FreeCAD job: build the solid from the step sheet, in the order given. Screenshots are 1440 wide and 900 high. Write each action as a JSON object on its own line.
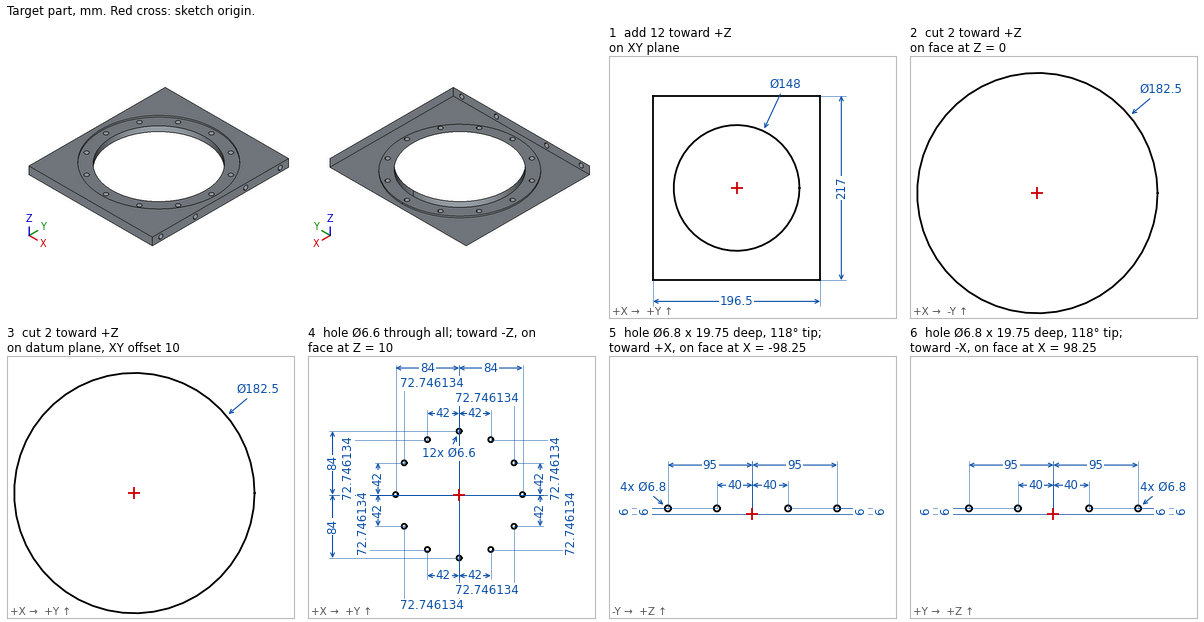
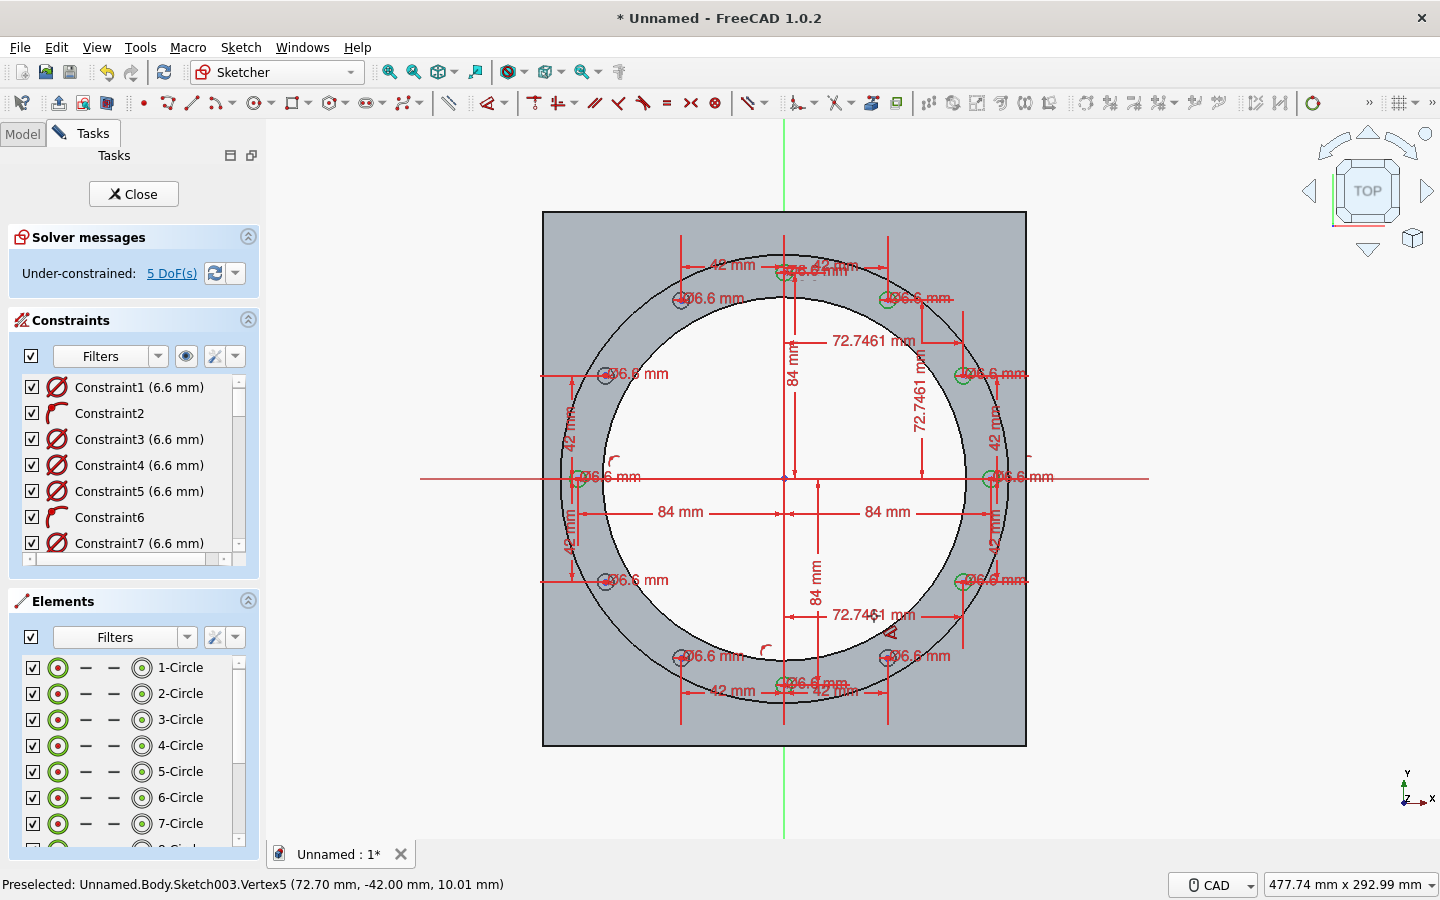
{"action": "left_click", "coordinate": [888, 658]}
{"action": "left_click", "coordinate": [922, 569]}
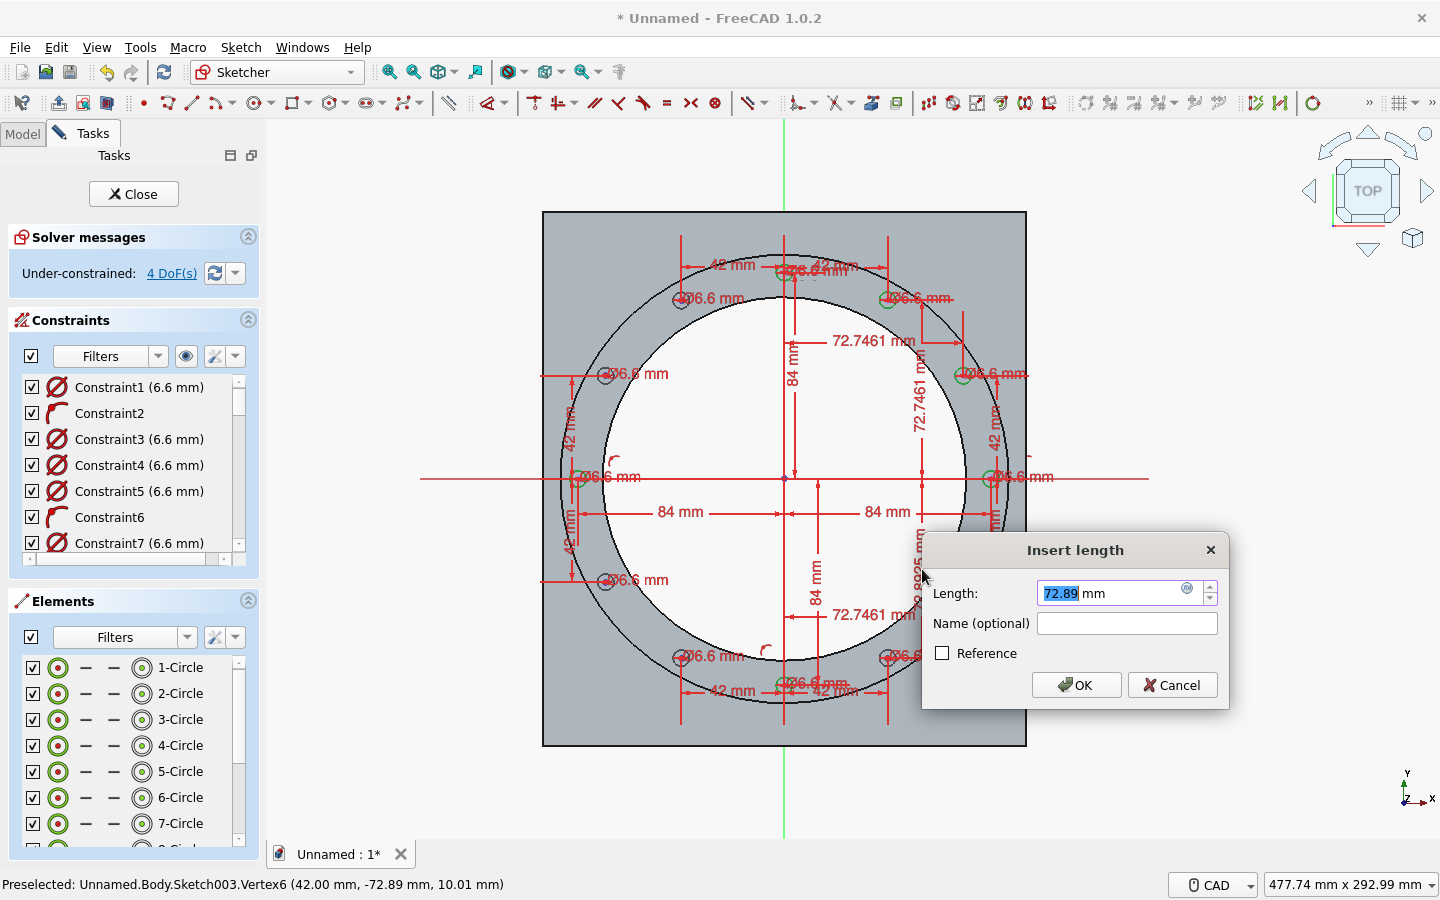
{"action": "type", "text": "72.746134"}
{"action": "key", "text": "Return"}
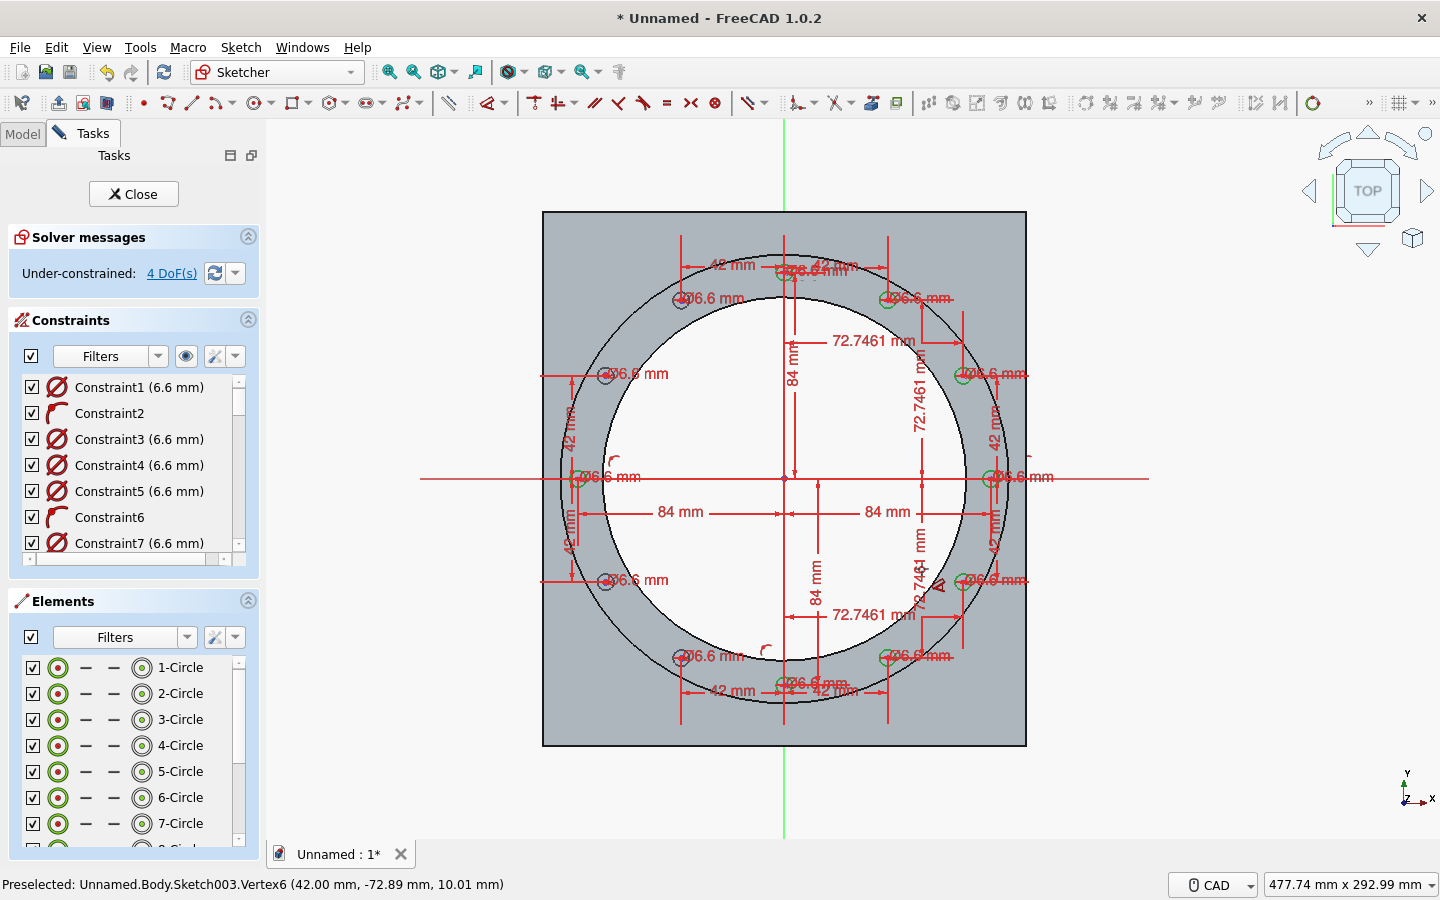
{"action": "left_click", "coordinate": [681, 658]}
{"action": "left_click", "coordinate": [647, 569]}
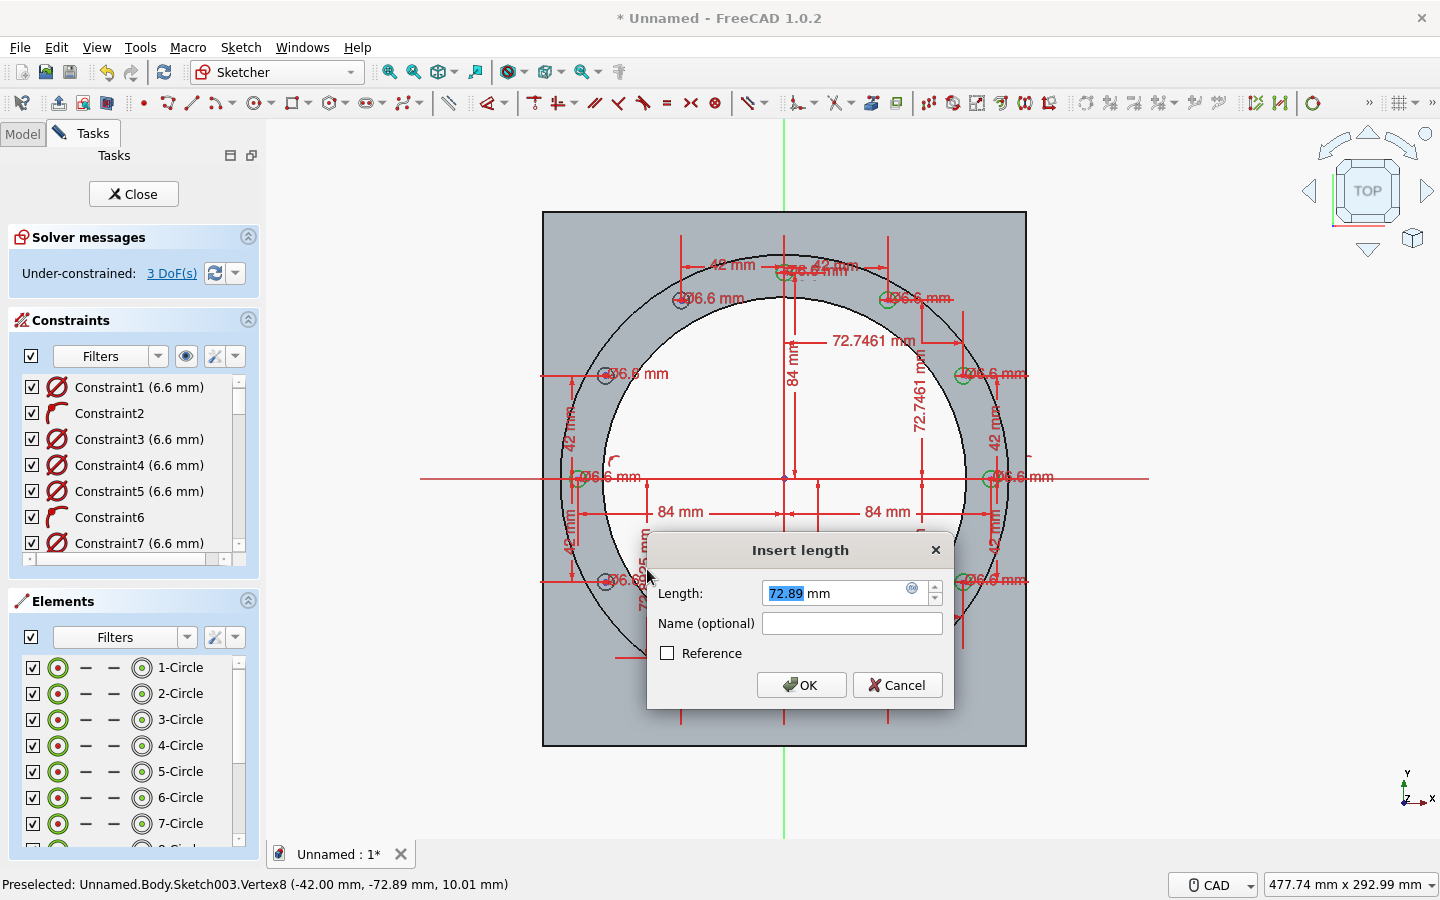
{"action": "type", "text": "72.746134"}
{"action": "key", "text": "Return"}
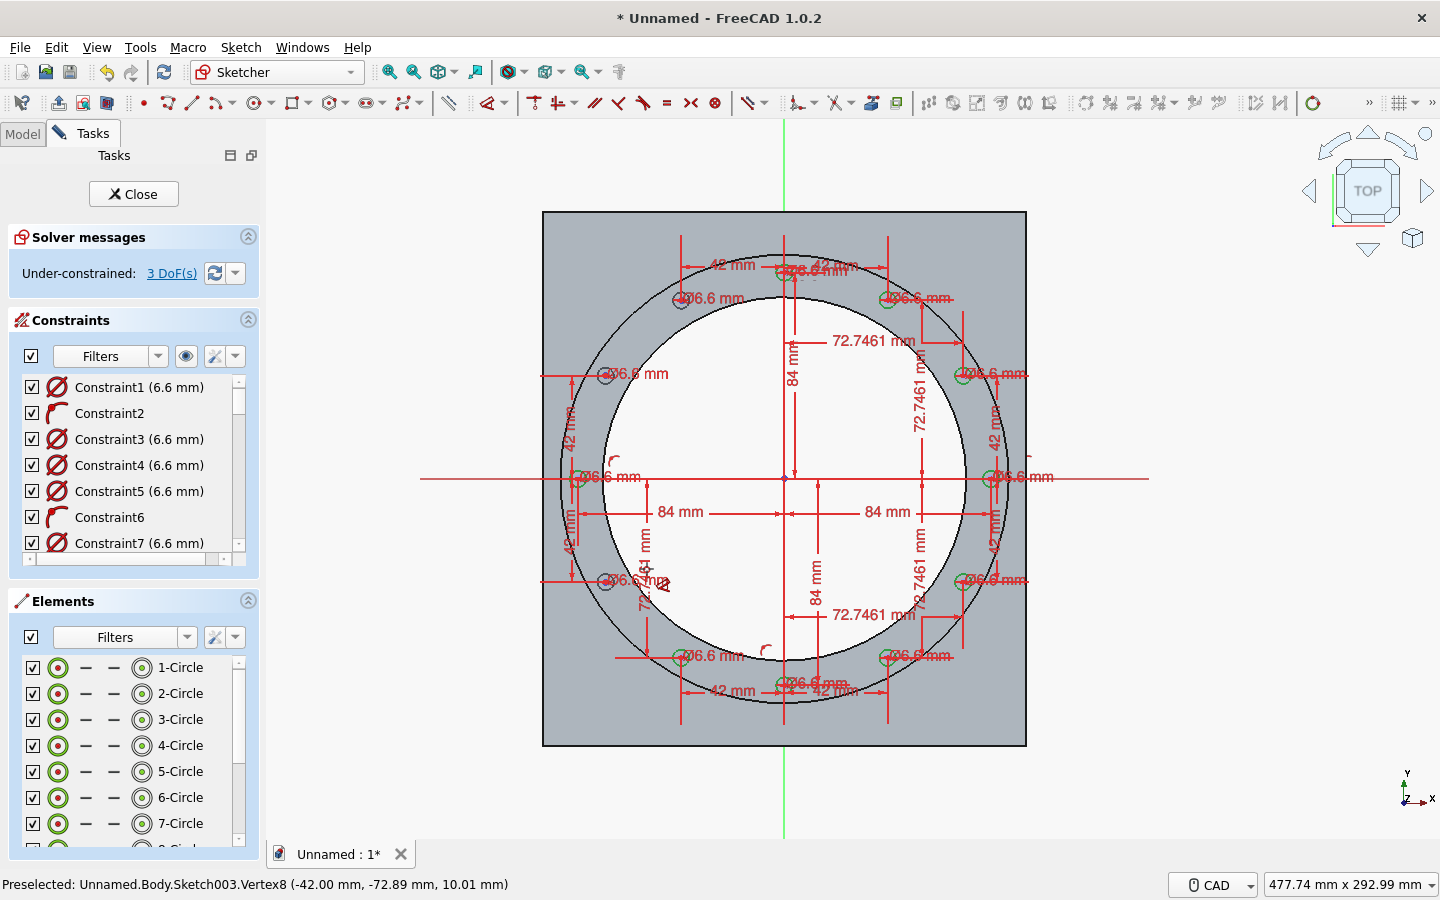
{"action": "left_click", "coordinate": [606, 582]}
{"action": "left_click", "coordinate": [695, 616]}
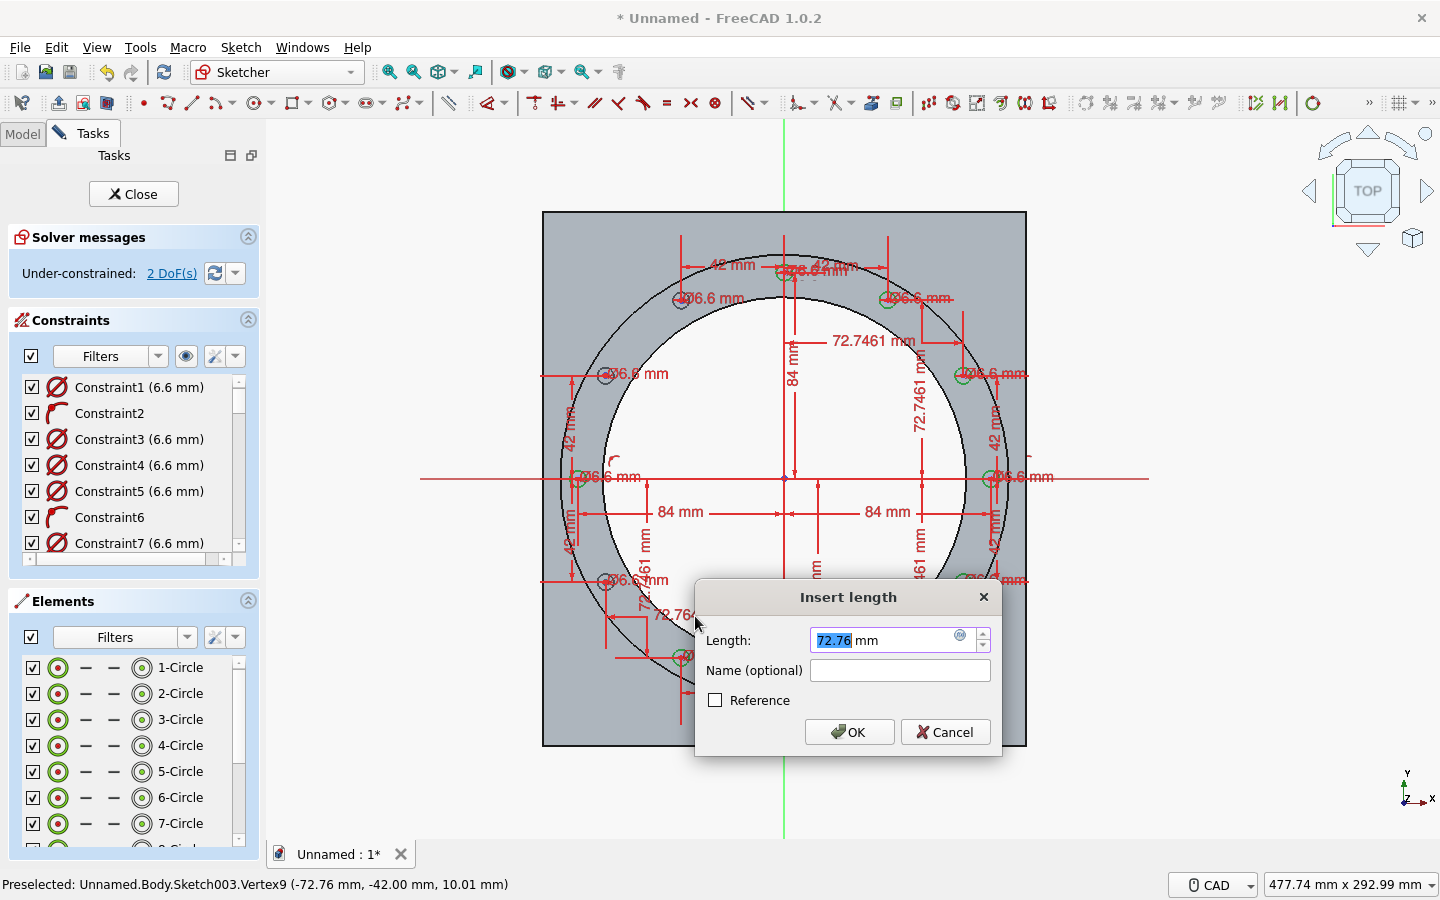
{"action": "type", "text": "72.746134"}
{"action": "key", "text": "Return"}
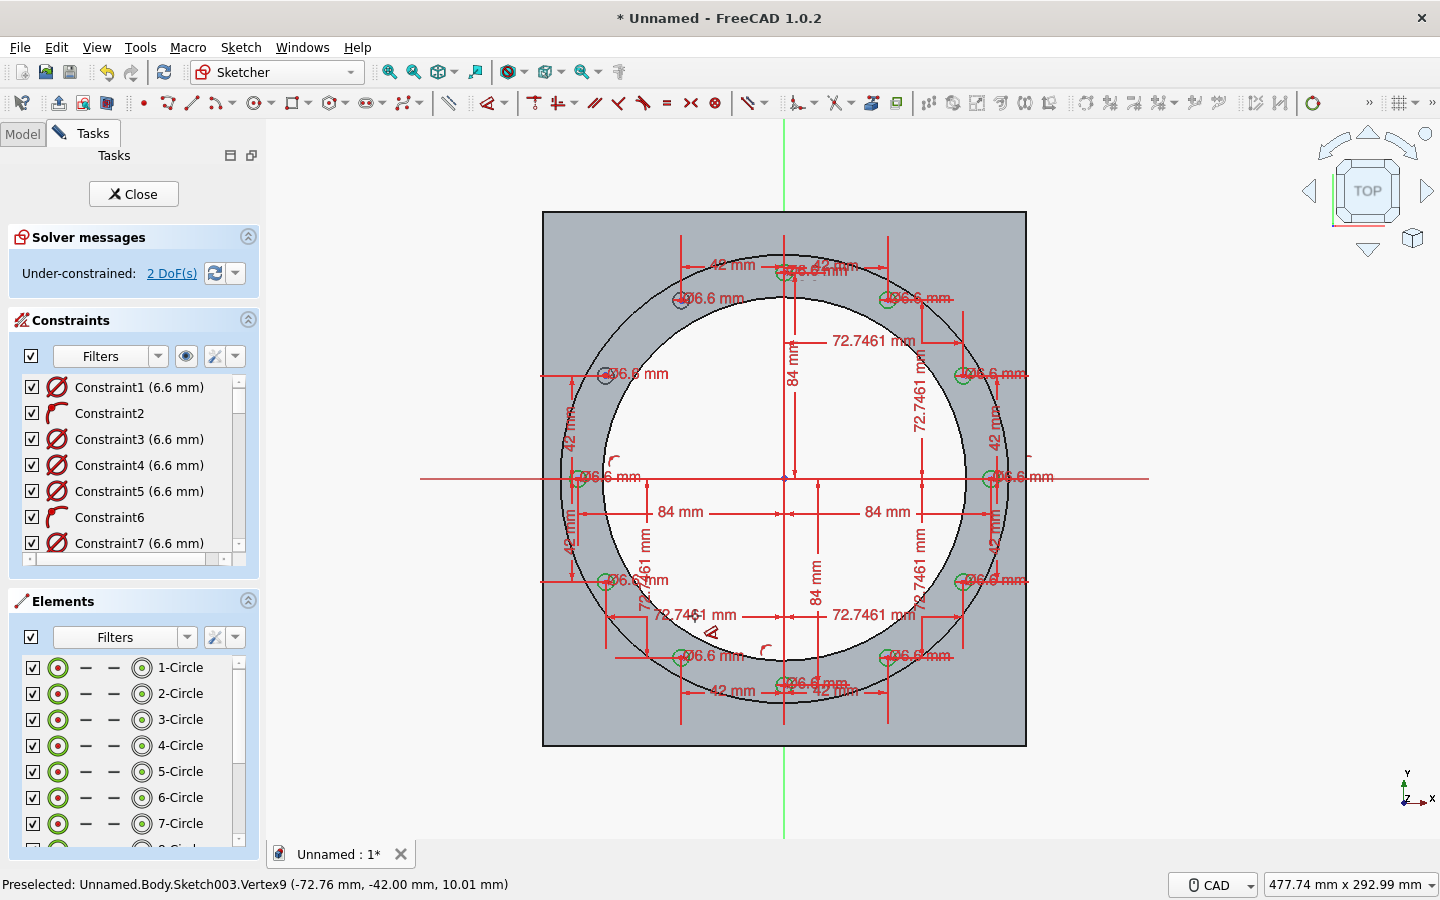
{"action": "left_click", "coordinate": [606, 376]}
{"action": "left_click", "coordinate": [695, 342]}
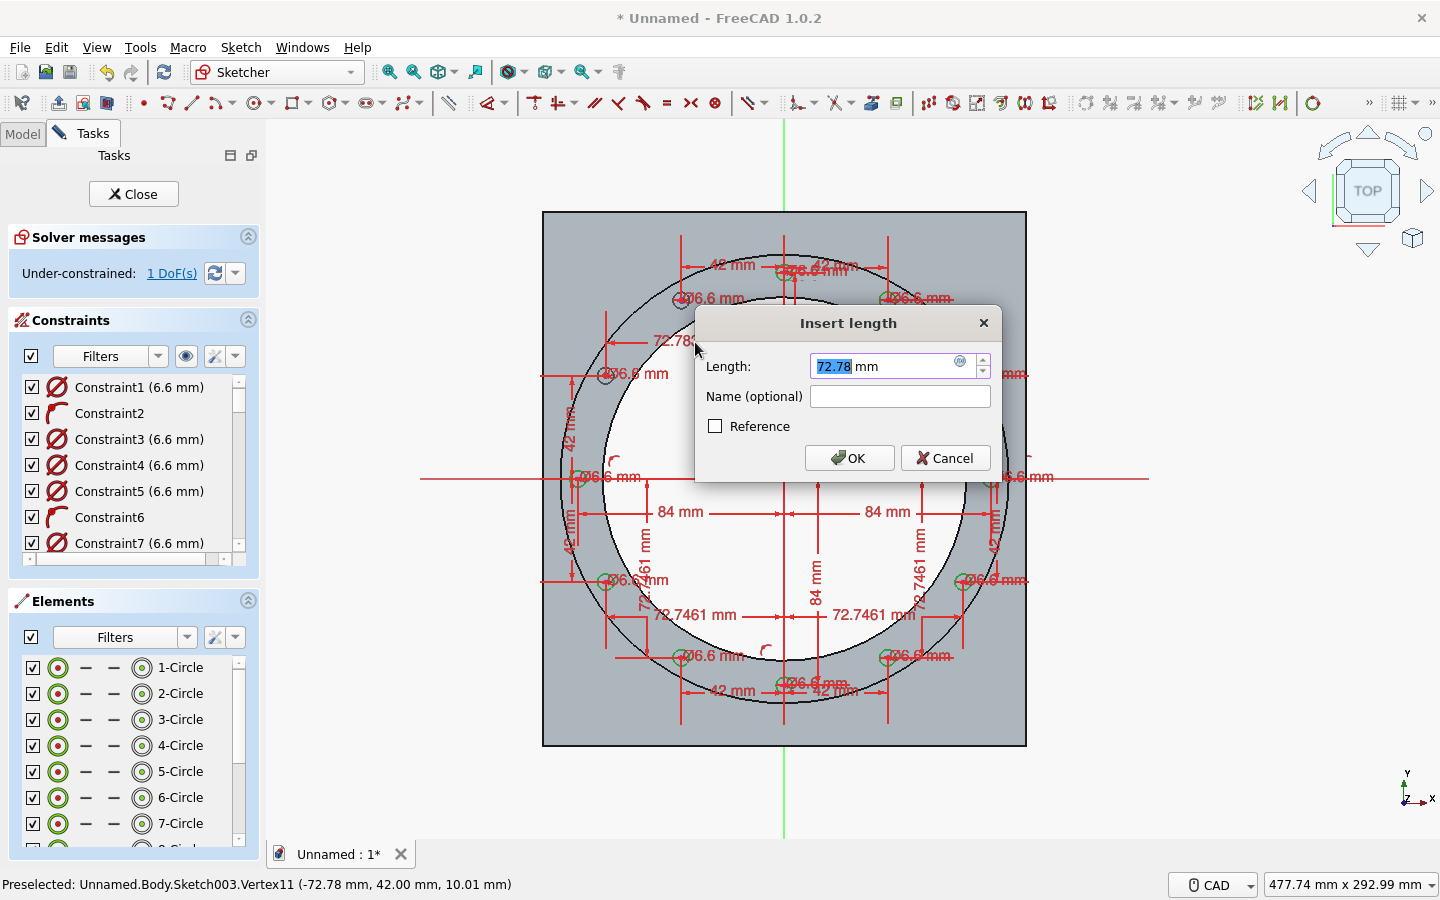
{"action": "type", "text": "72.746134"}
{"action": "key", "text": "Return"}